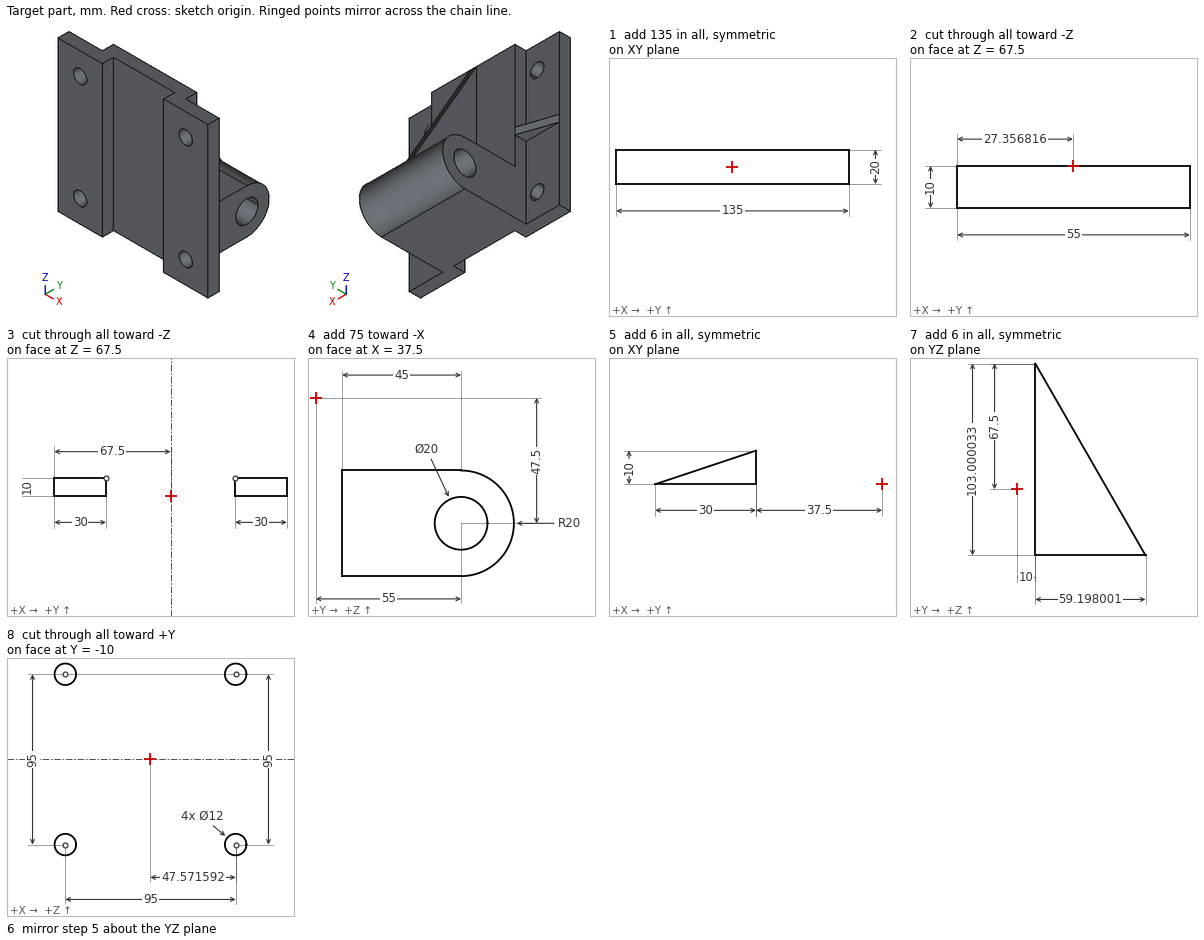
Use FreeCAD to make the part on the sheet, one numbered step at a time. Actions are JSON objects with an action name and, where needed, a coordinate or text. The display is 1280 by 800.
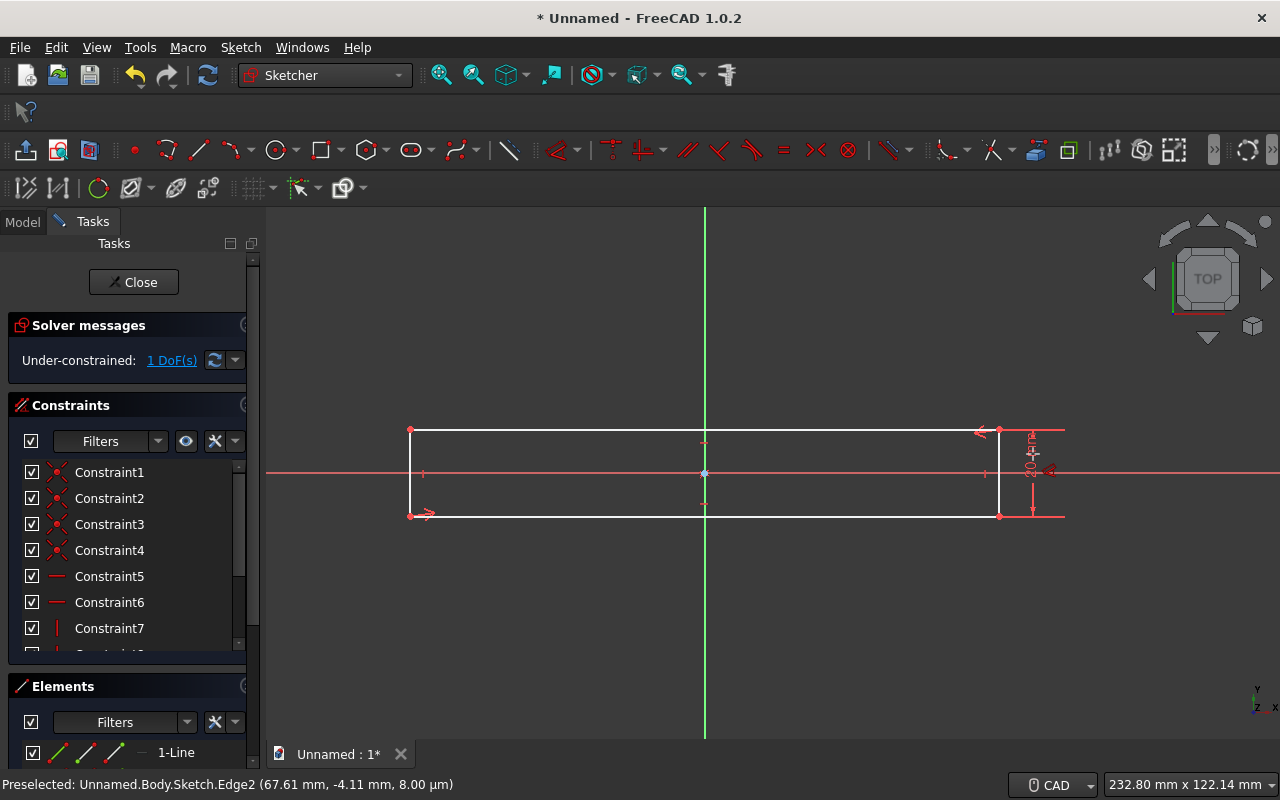
{"action": "left_click", "coordinate": [587, 517]}
{"action": "left_click", "coordinate": [569, 551]}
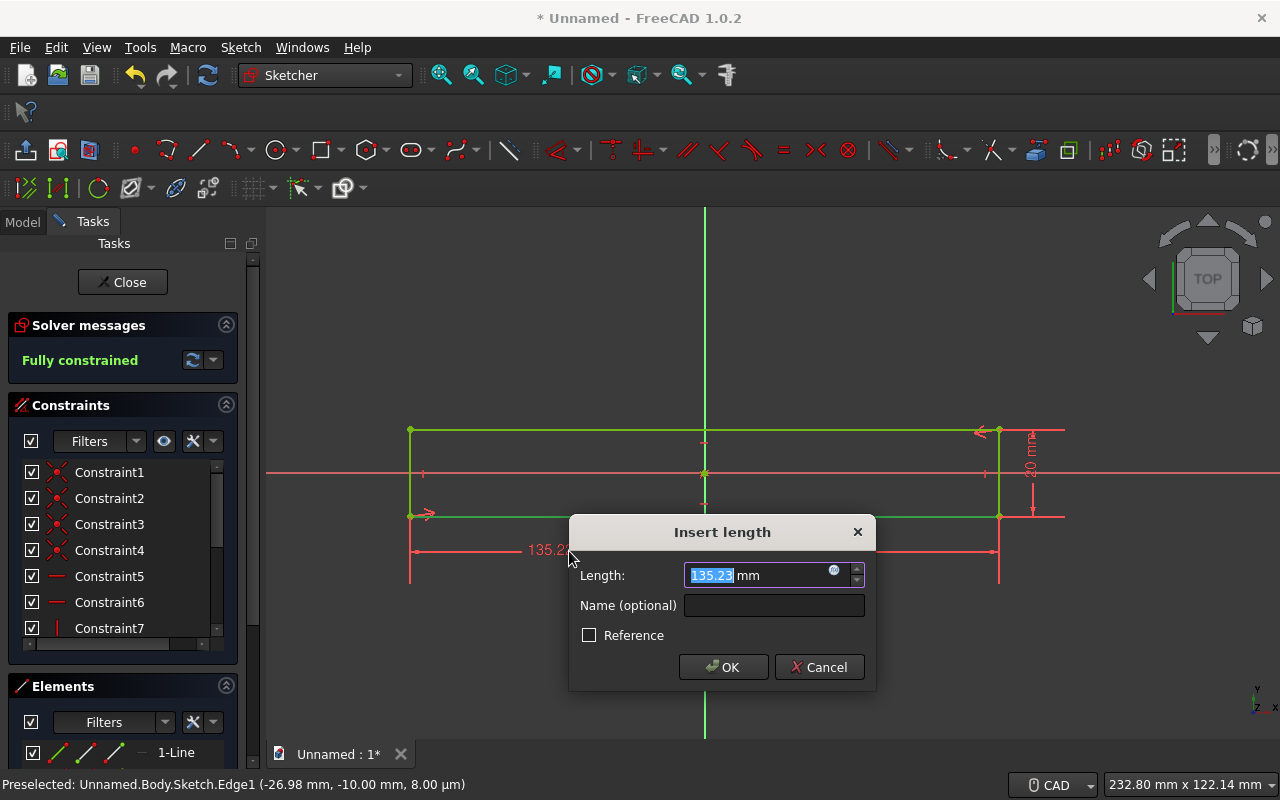
{"action": "type", "text": "135"}
{"action": "key", "text": "Return"}
{"action": "key", "text": "Escape"}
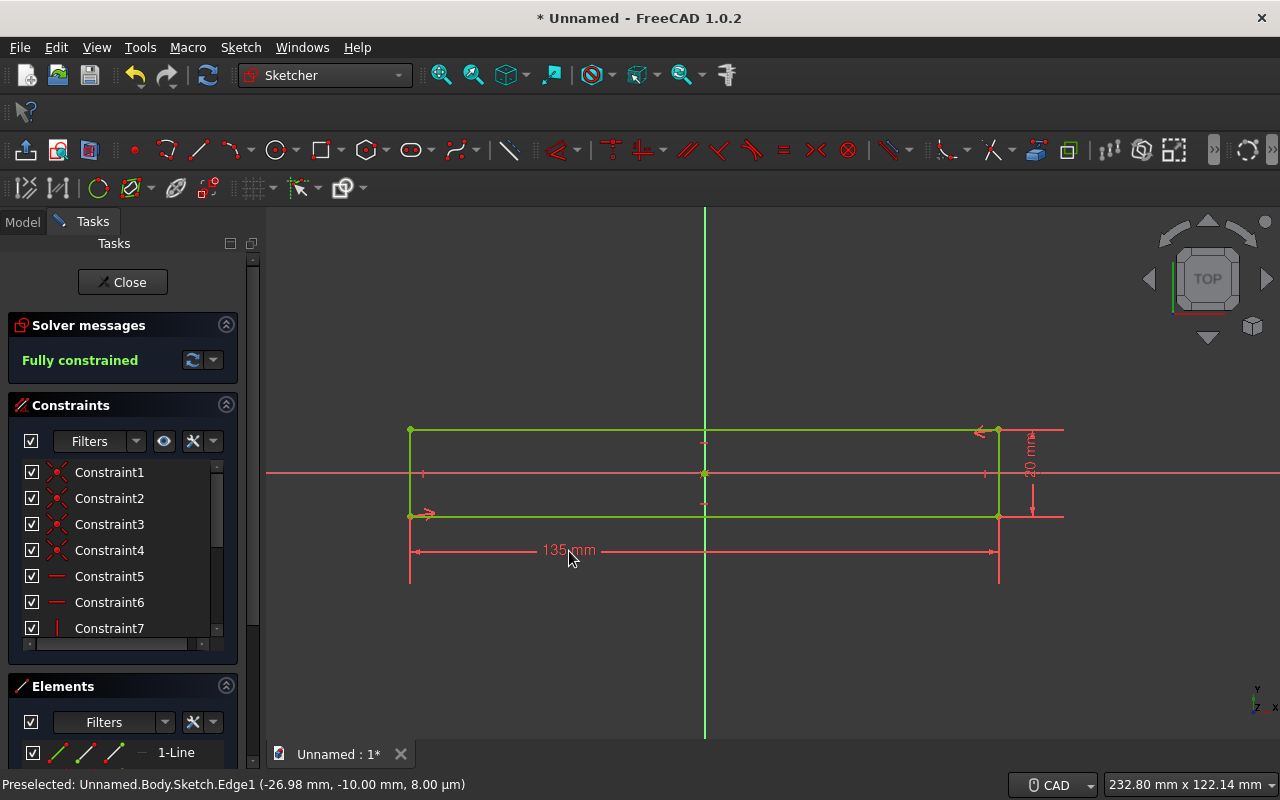
{"action": "left_click", "coordinate": [123, 282]}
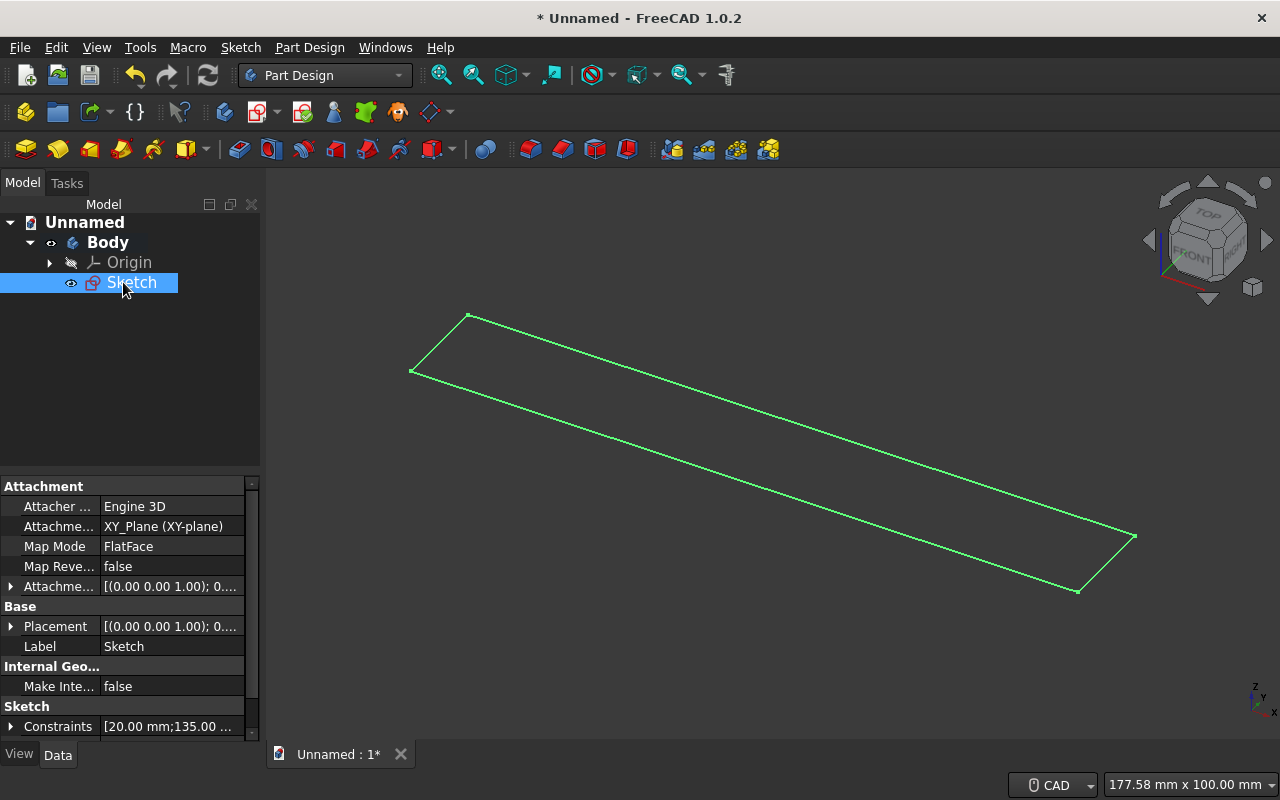
{"action": "left_click", "coordinate": [26, 150]}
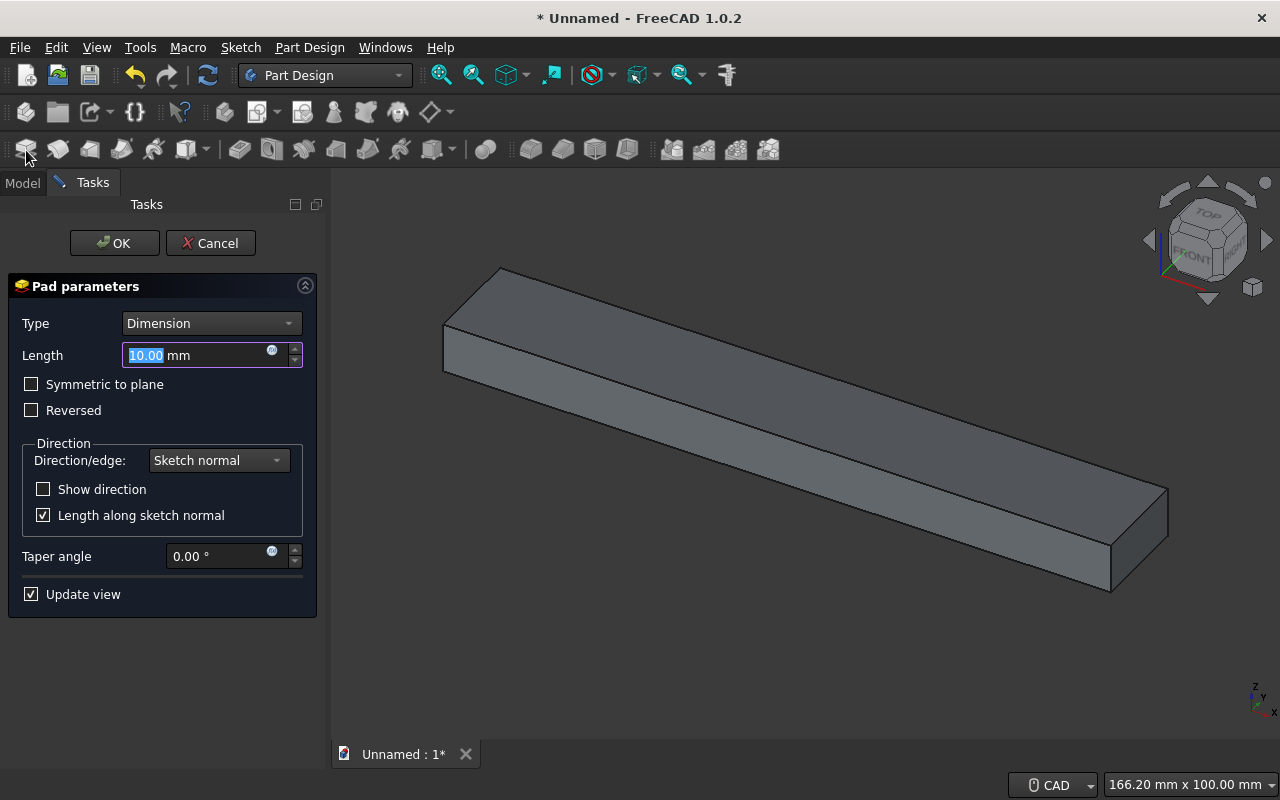
{"action": "type", "text": "135"}
{"action": "key", "text": "Tab"}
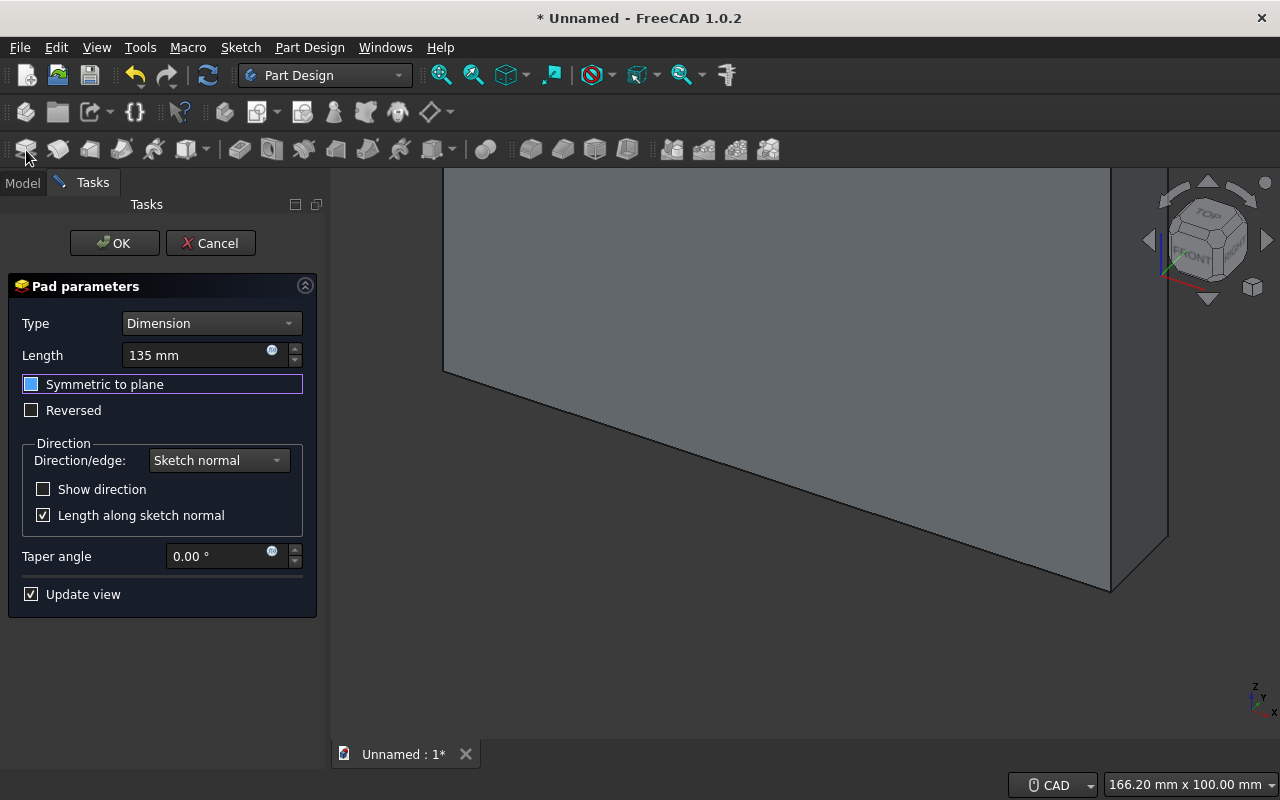
{"action": "left_click", "coordinate": [30, 384]}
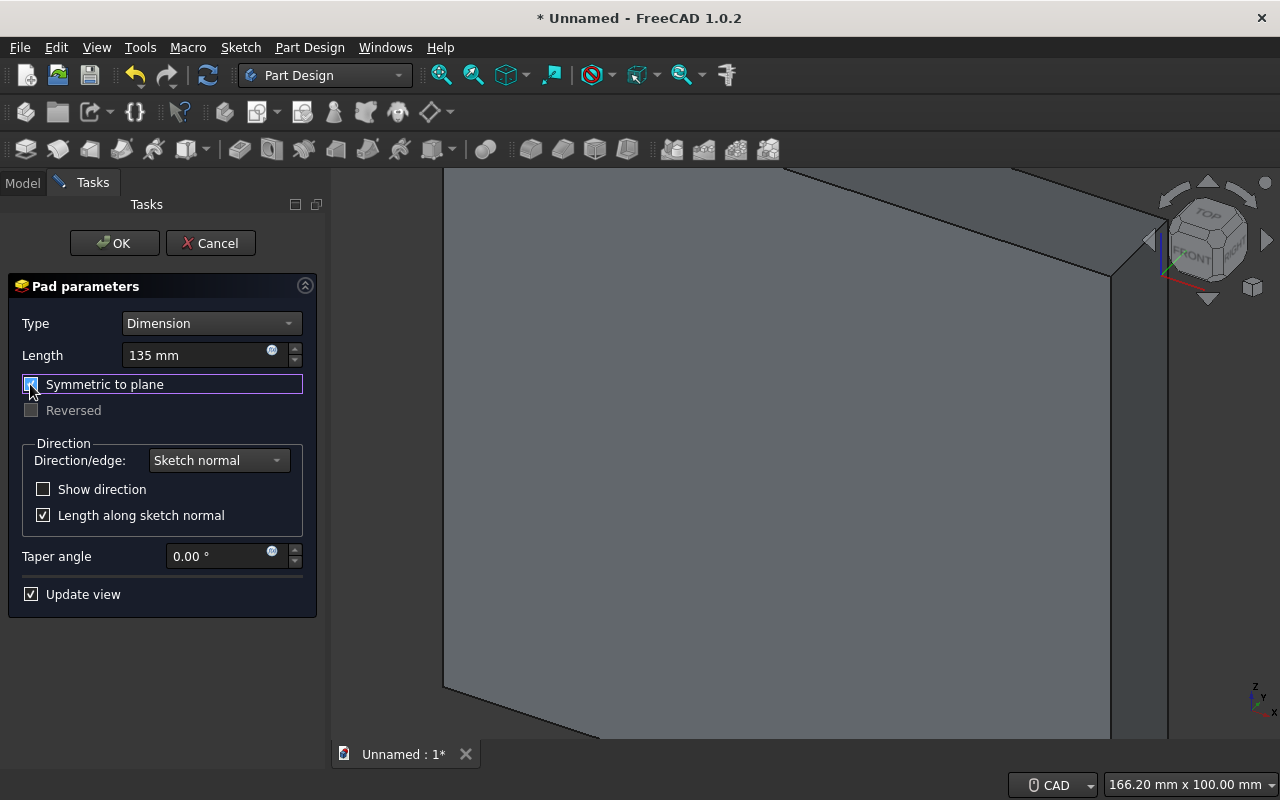
{"action": "left_click", "coordinate": [115, 243]}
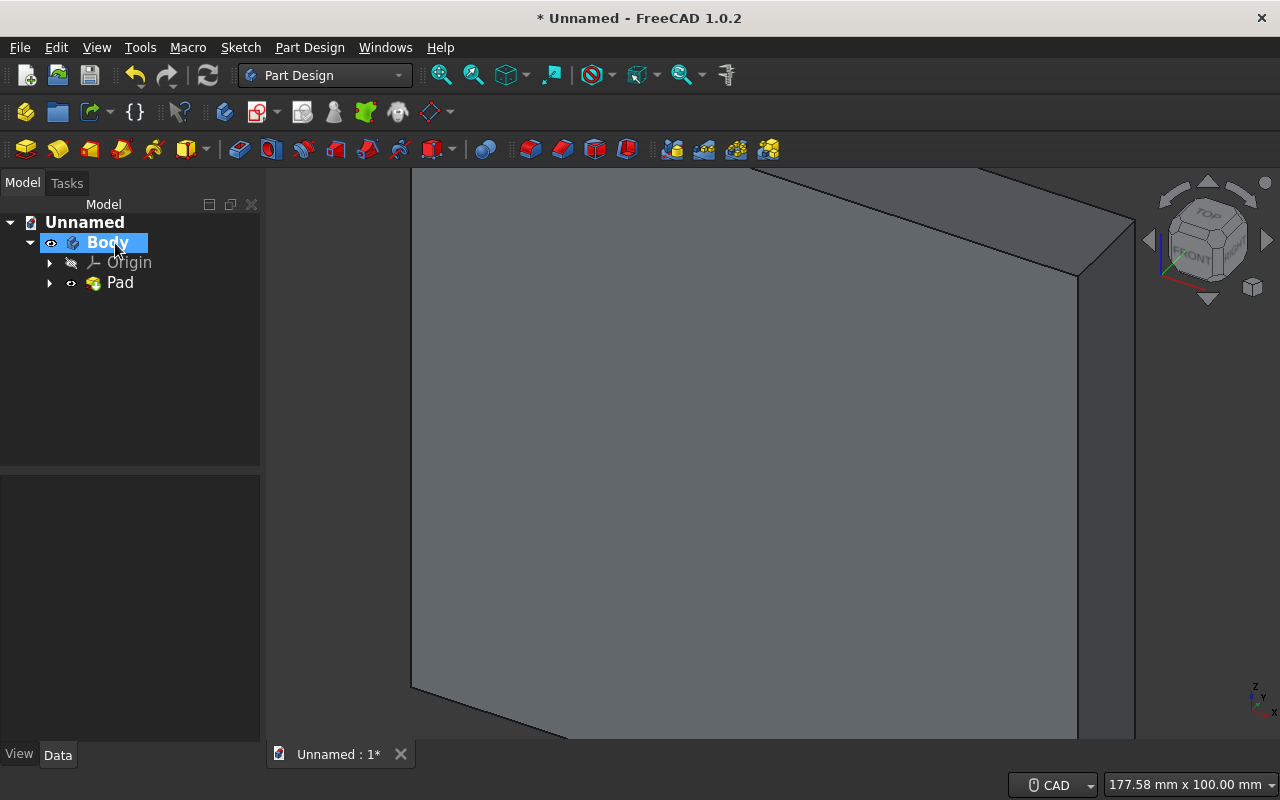
{"action": "key", "text": "v f"}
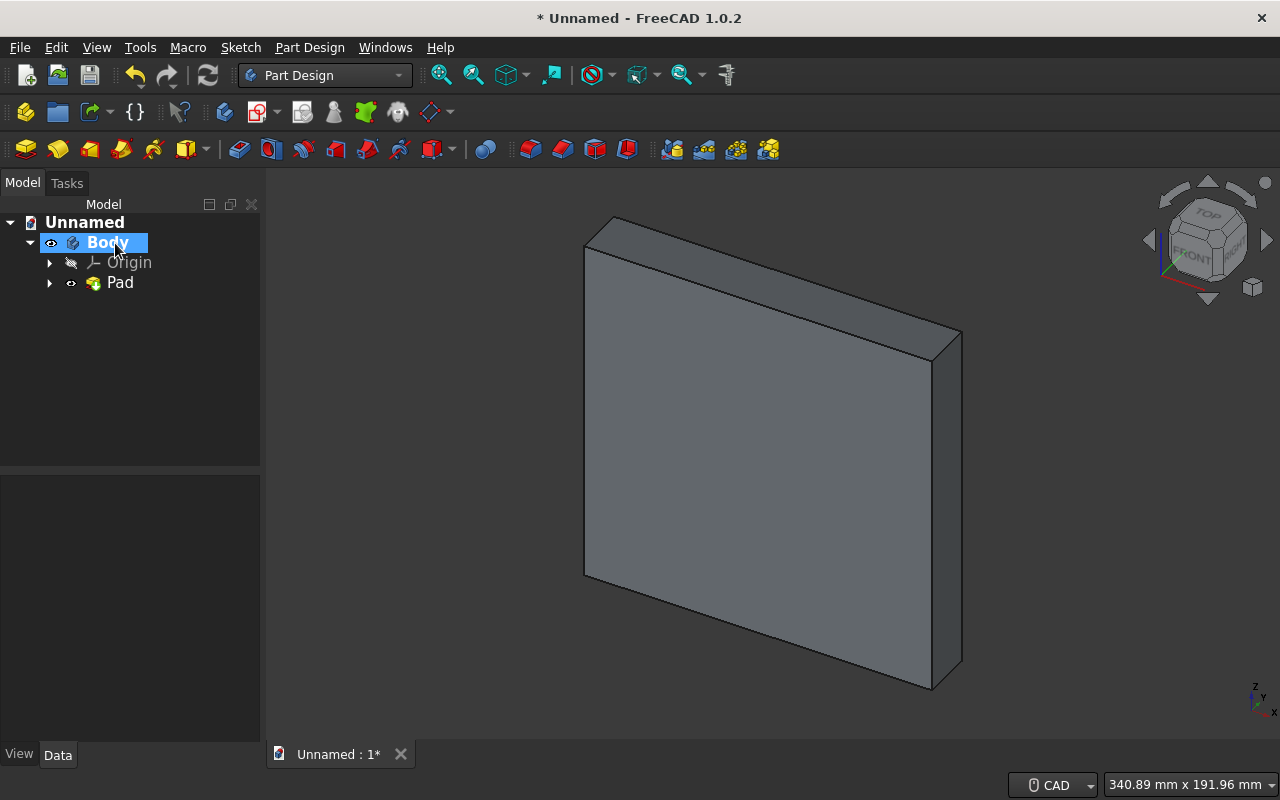
{"action": "left_click", "coordinate": [872, 321]}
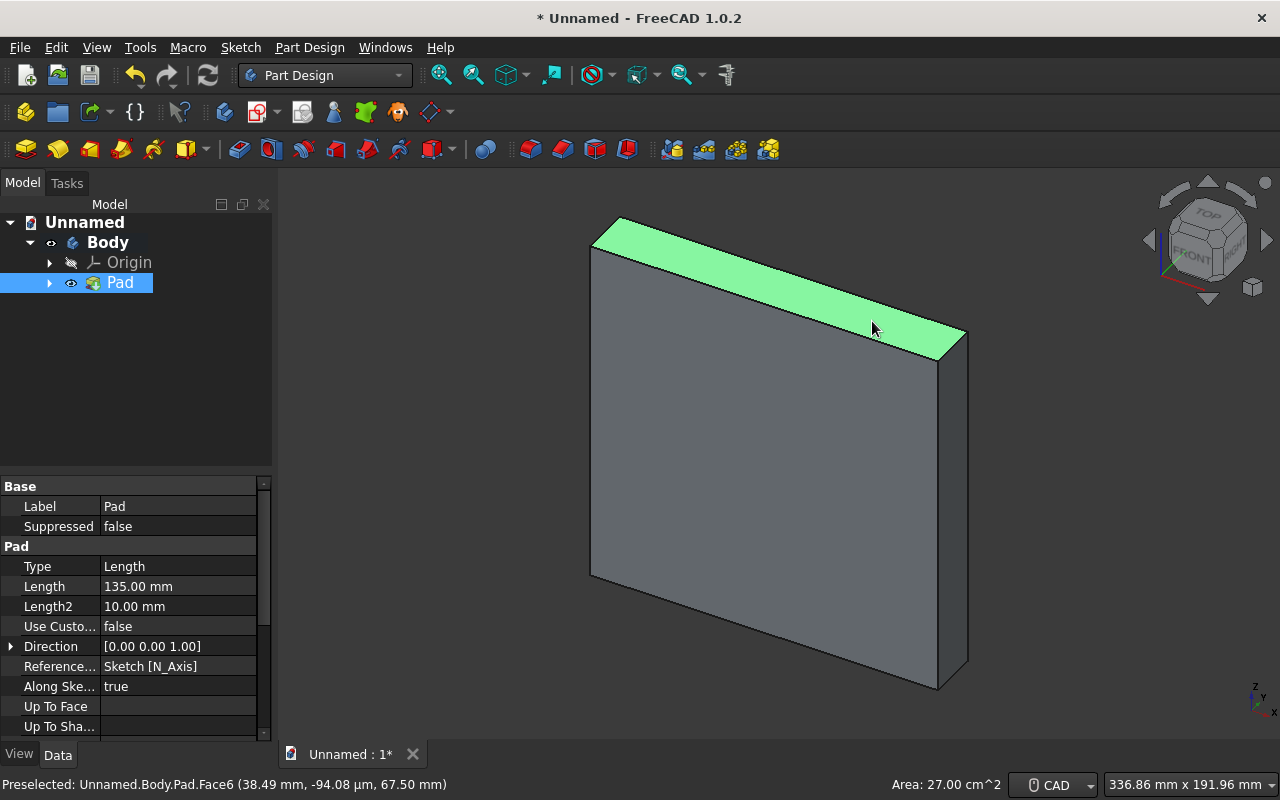
{"action": "left_click", "coordinate": [258, 112]}